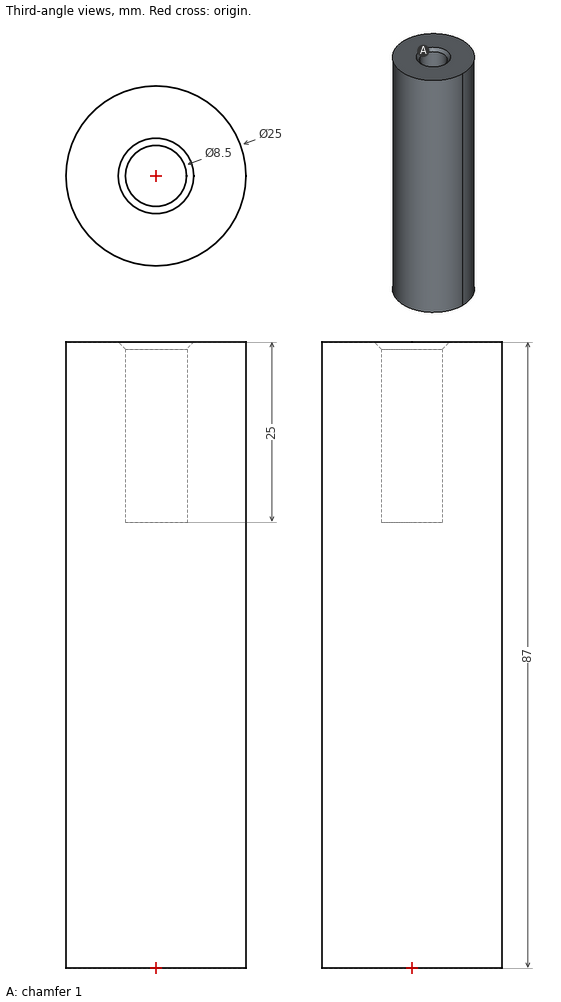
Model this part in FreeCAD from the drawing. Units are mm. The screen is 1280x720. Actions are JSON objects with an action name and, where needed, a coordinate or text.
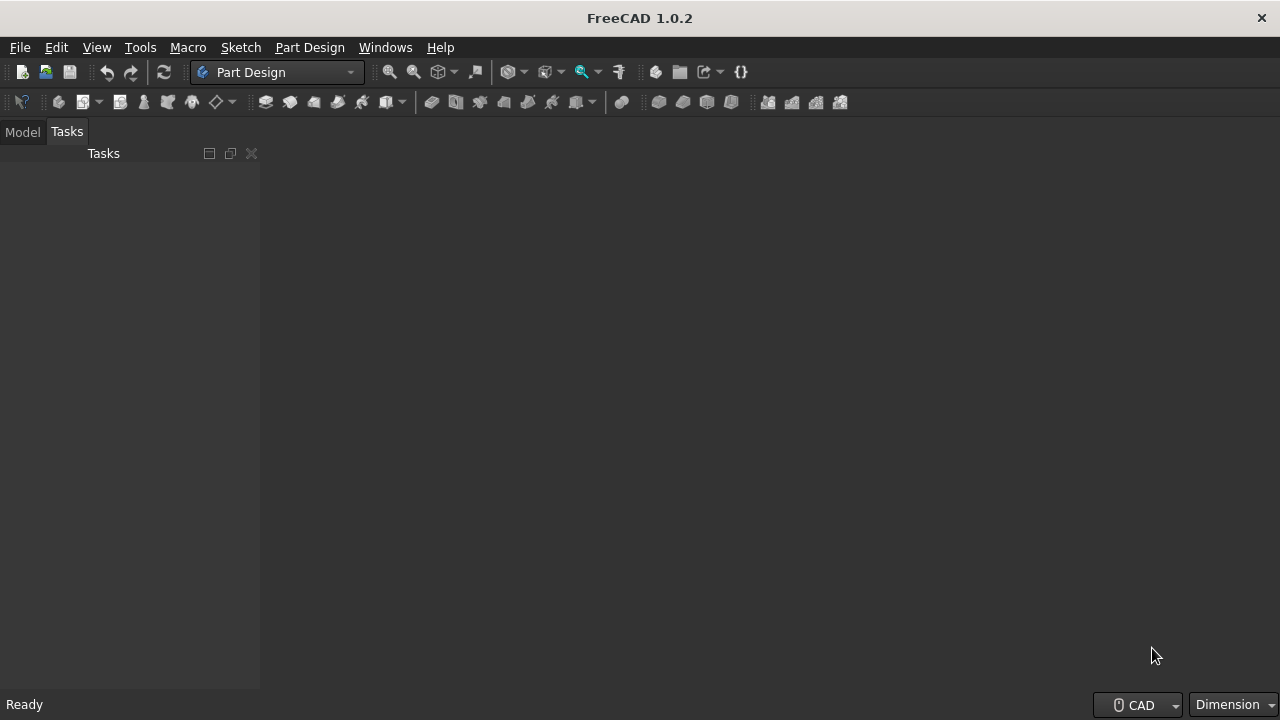
{"action": "key", "text": "ctrl+n"}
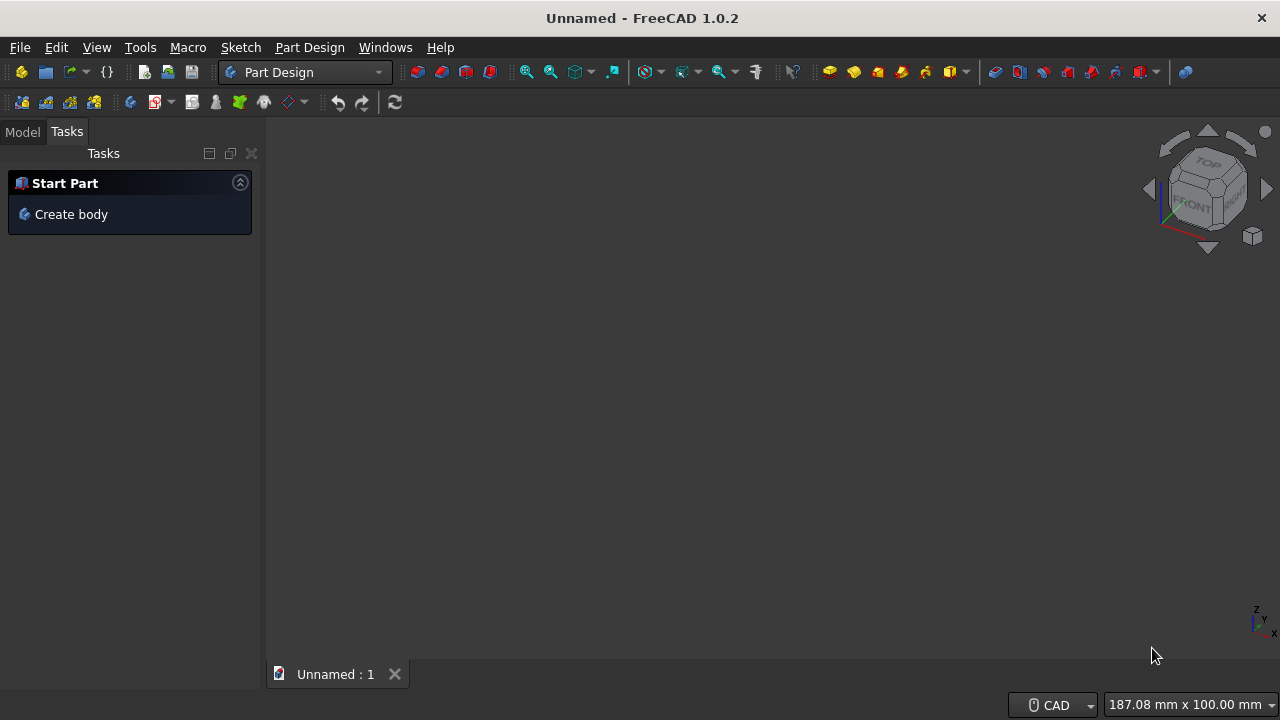
{"action": "left_click", "coordinate": [156, 102]}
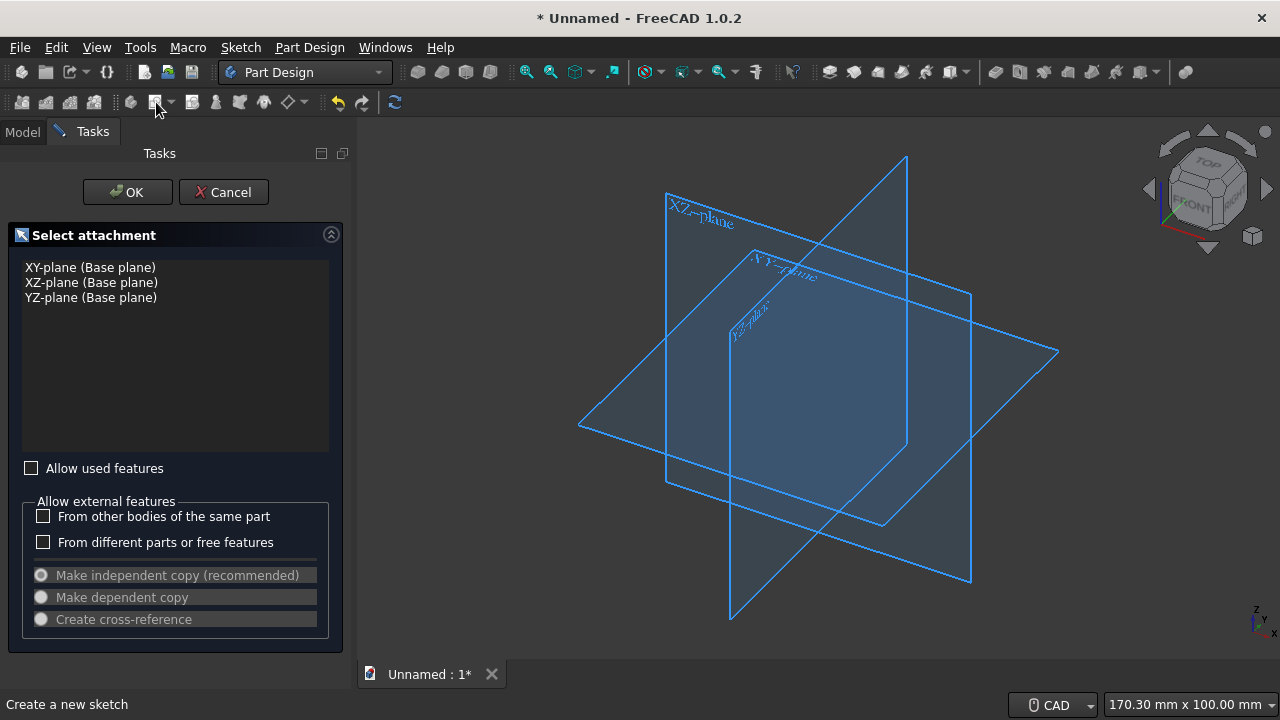
{"action": "left_click", "coordinate": [82, 268]}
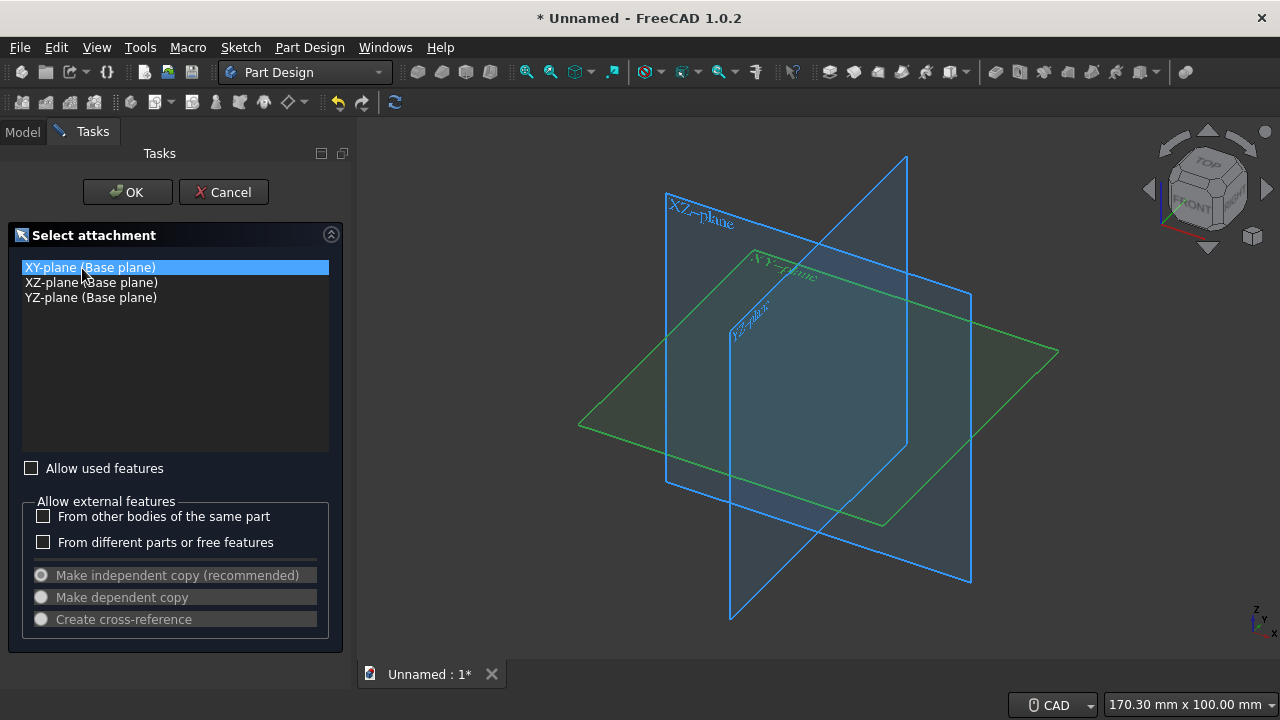
{"action": "left_click", "coordinate": [128, 192]}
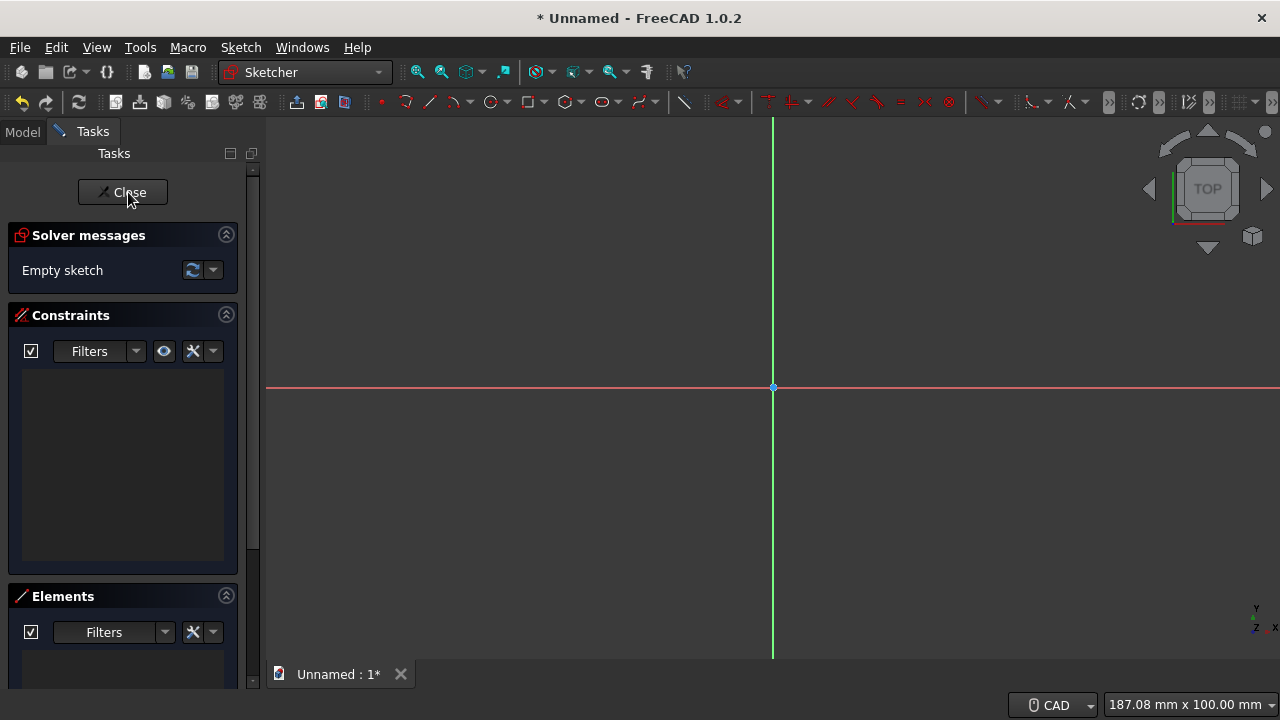
{"action": "scroll", "coordinate": [813, 388], "scroll_direction": "up", "scroll_amount": 5}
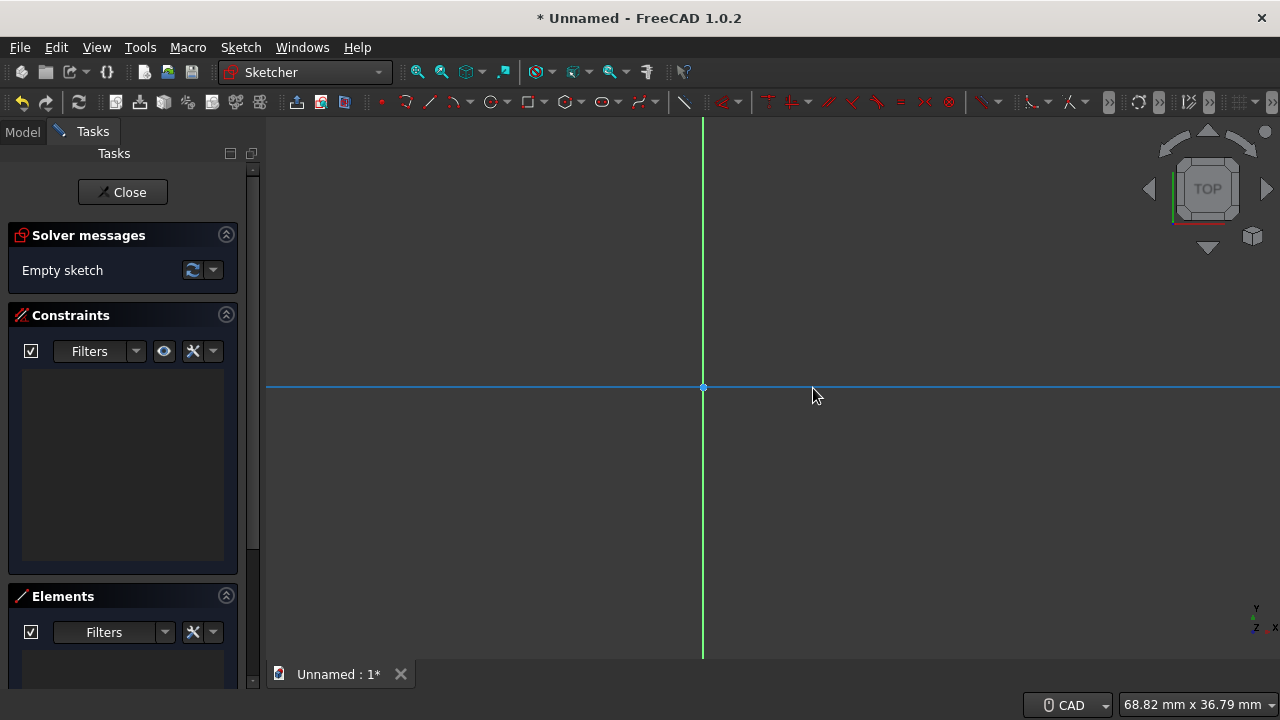
{"action": "left_click", "coordinate": [492, 102]}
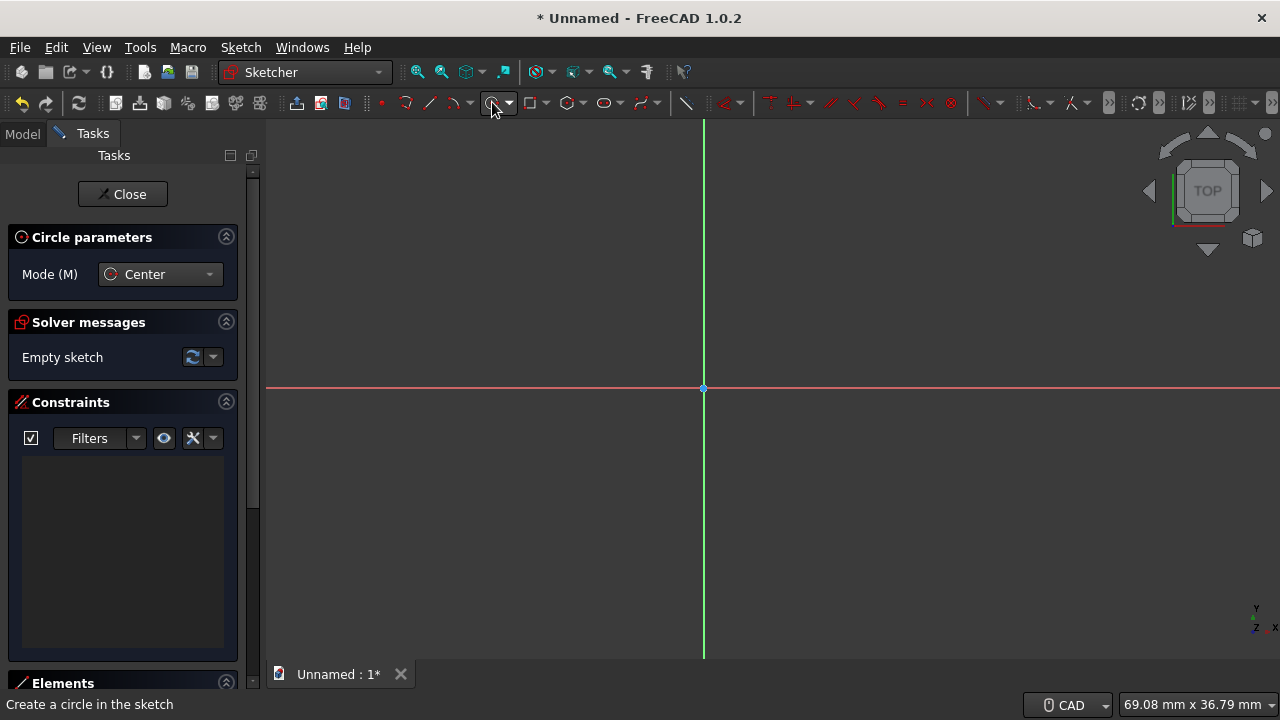
{"action": "left_click", "coordinate": [704, 388]}
{"action": "left_click", "coordinate": [833, 258]}
{"action": "key", "text": "Escape"}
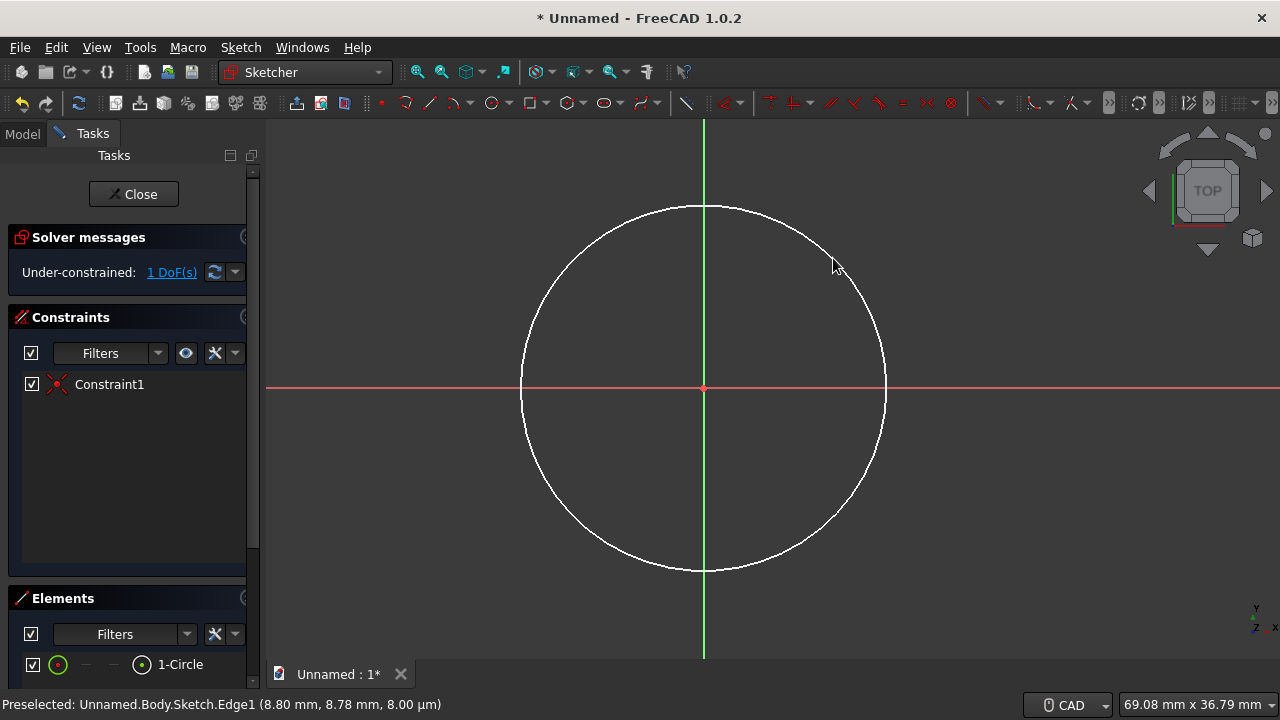
{"action": "left_click", "coordinate": [724, 104]}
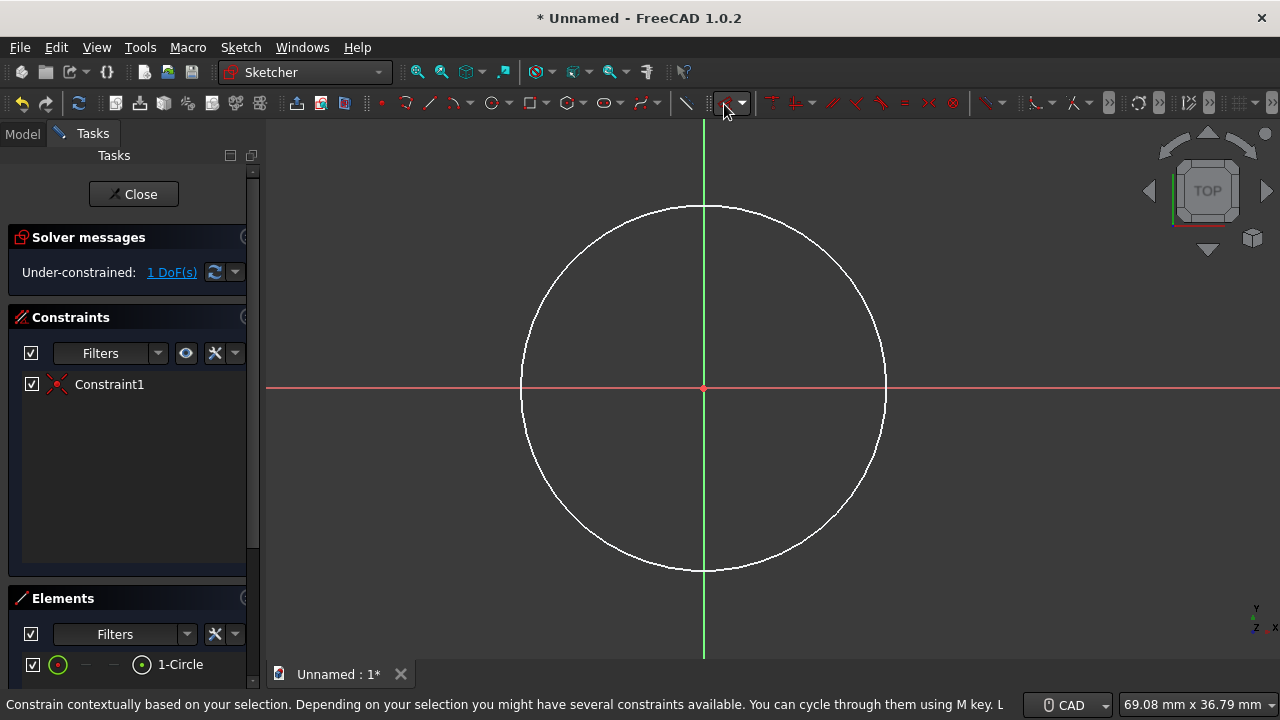
{"action": "left_click", "coordinate": [832, 258]}
{"action": "left_click", "coordinate": [854, 235]}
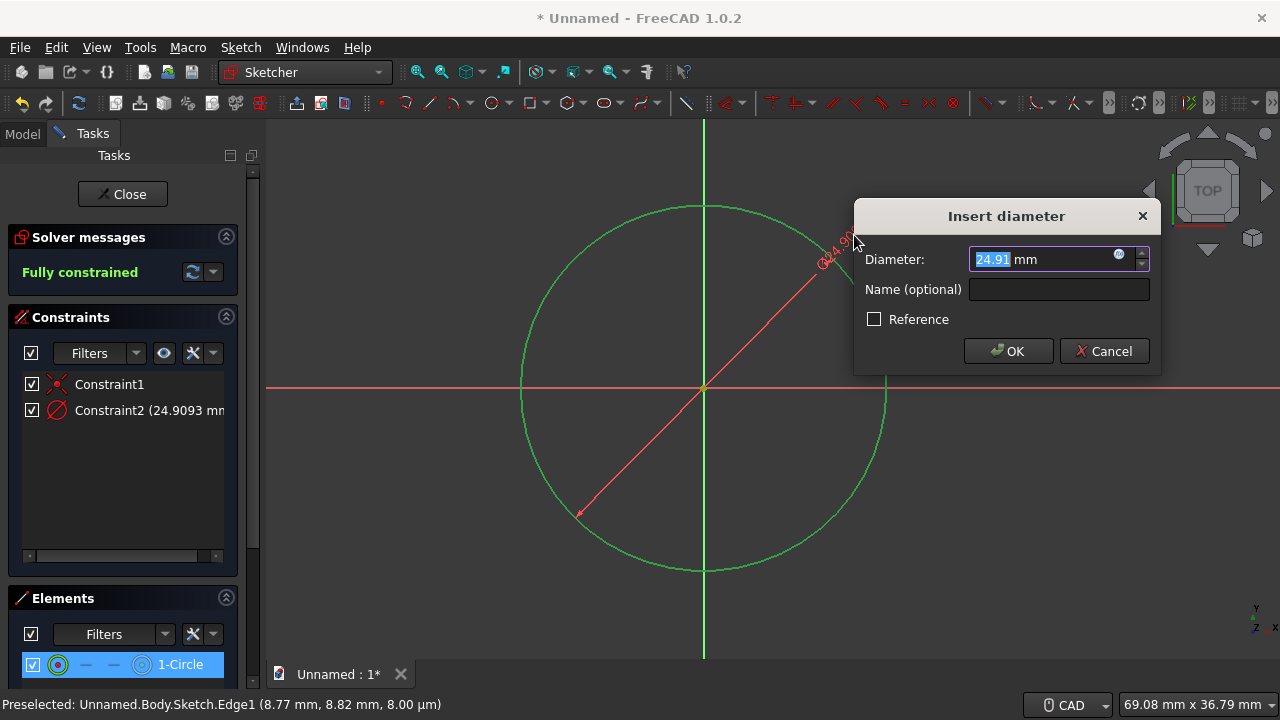
{"action": "type", "text": "25"}
{"action": "key", "text": "Return"}
{"action": "key", "text": "Escape"}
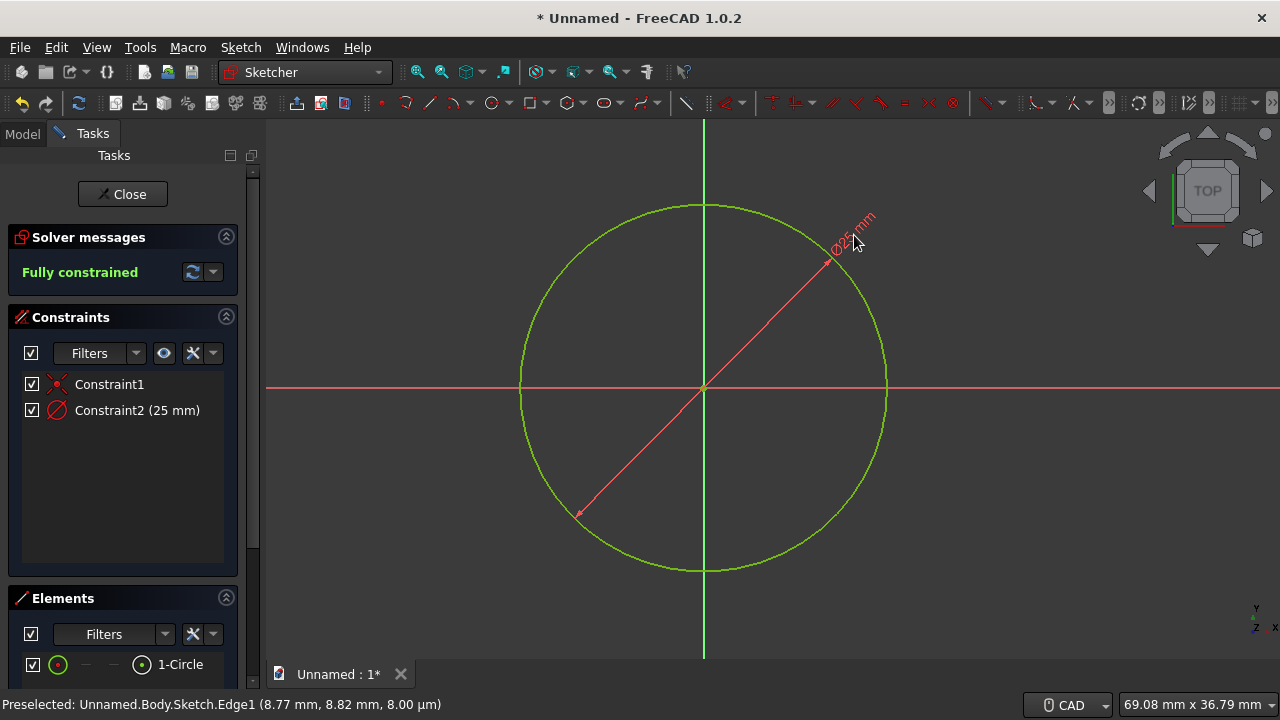
{"action": "left_click", "coordinate": [123, 194]}